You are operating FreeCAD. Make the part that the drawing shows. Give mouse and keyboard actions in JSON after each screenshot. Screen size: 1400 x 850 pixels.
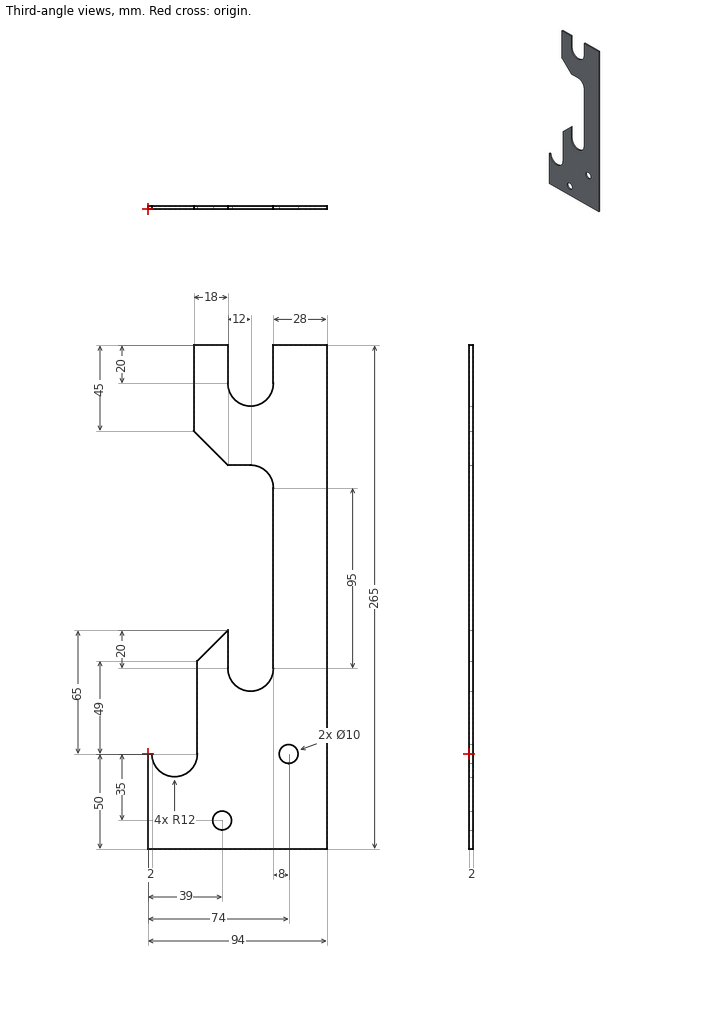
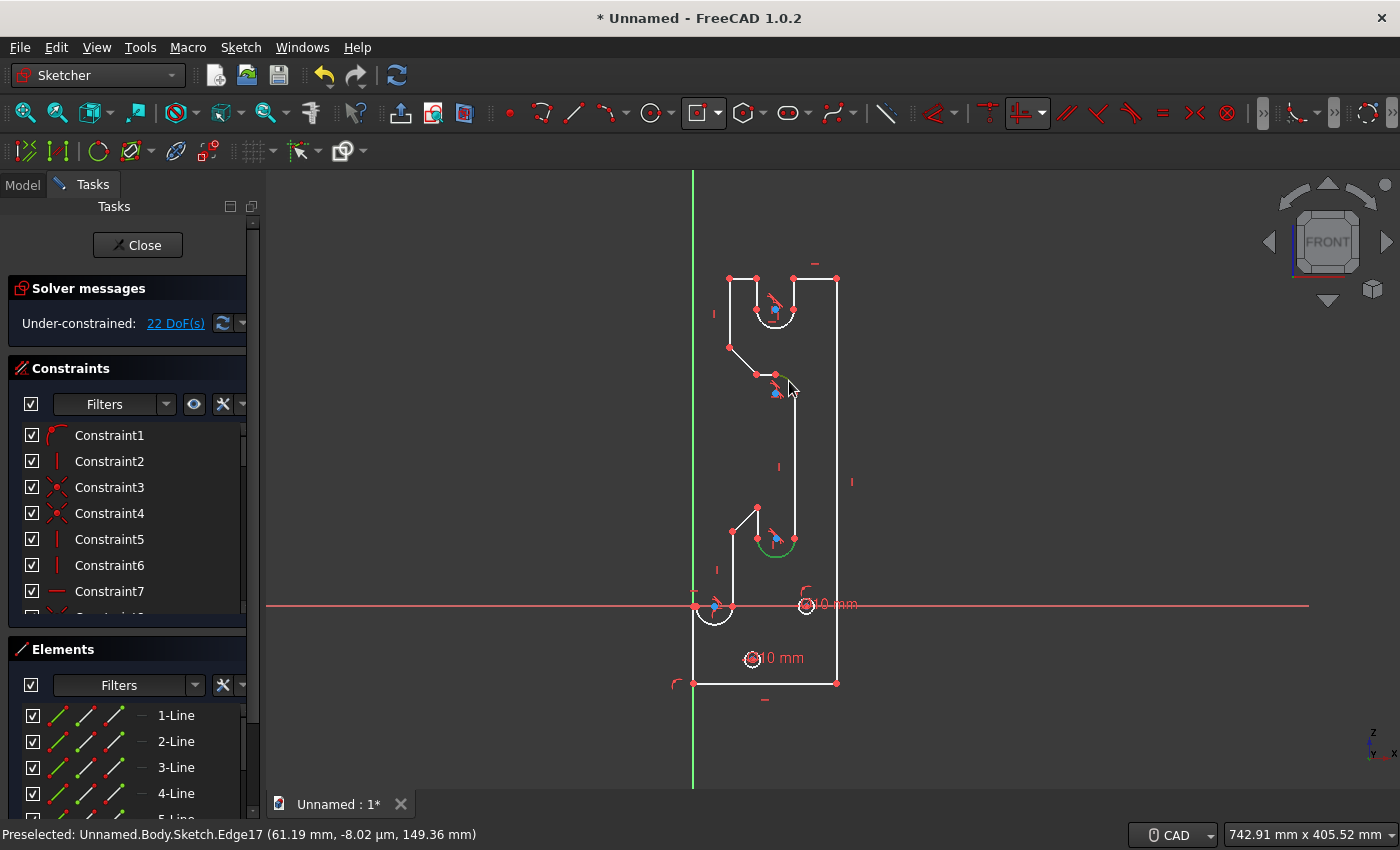
{"action": "left_click", "coordinate": [765, 325]}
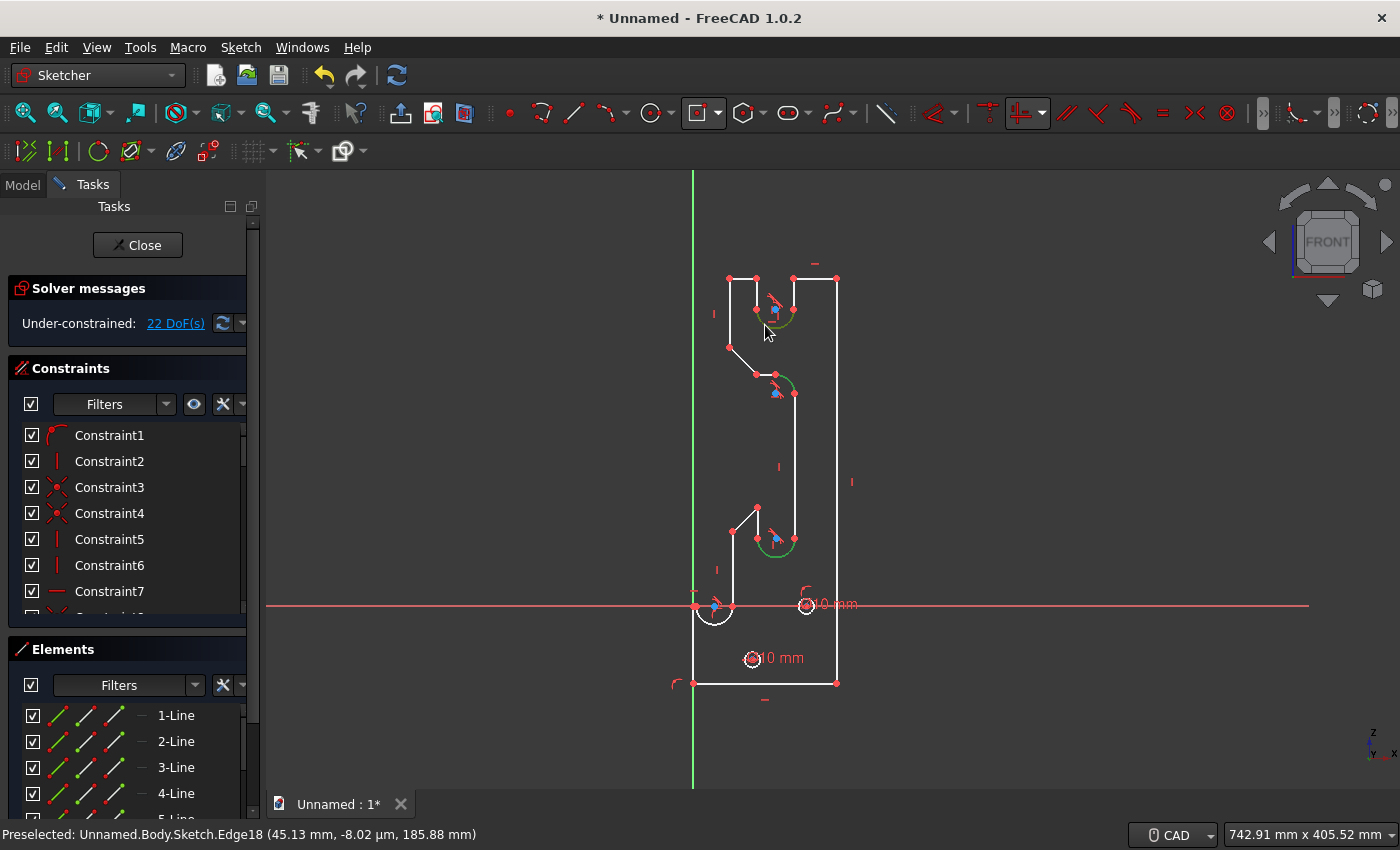
{"action": "scroll", "coordinate": [704, 621], "scroll_direction": "up", "scroll_amount": 2}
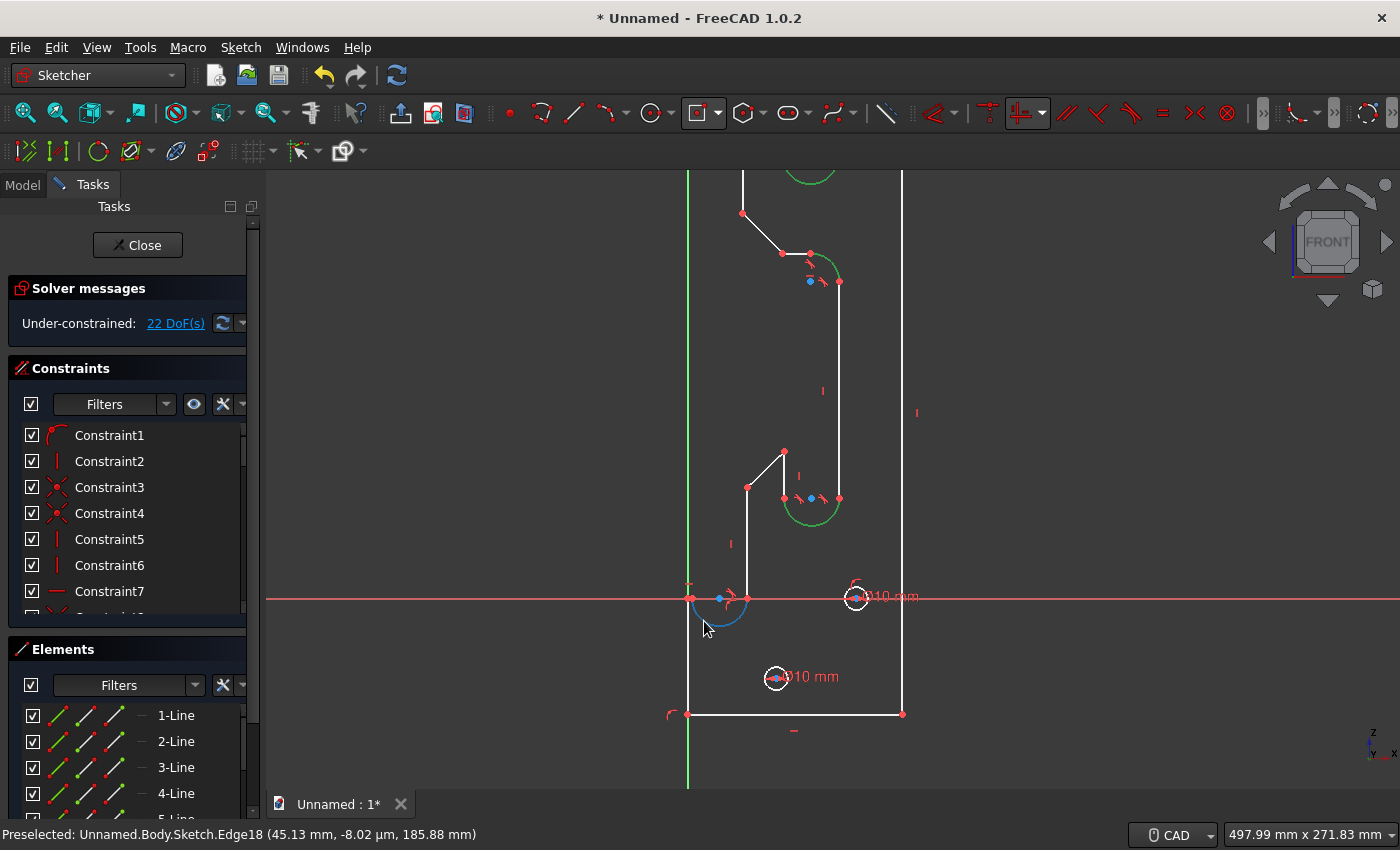
{"action": "left_click", "coordinate": [703, 621]}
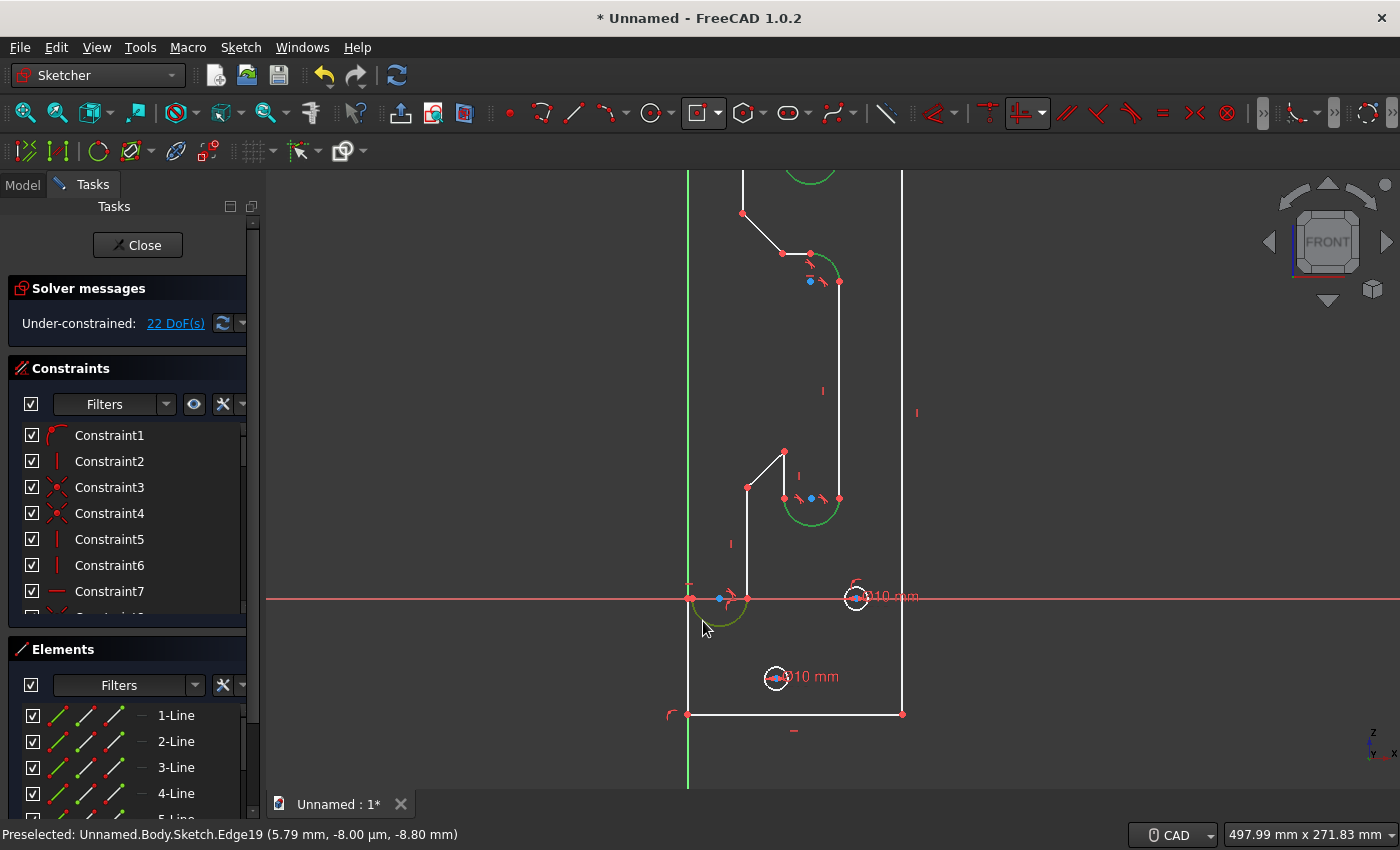
{"action": "key", "text": "e"}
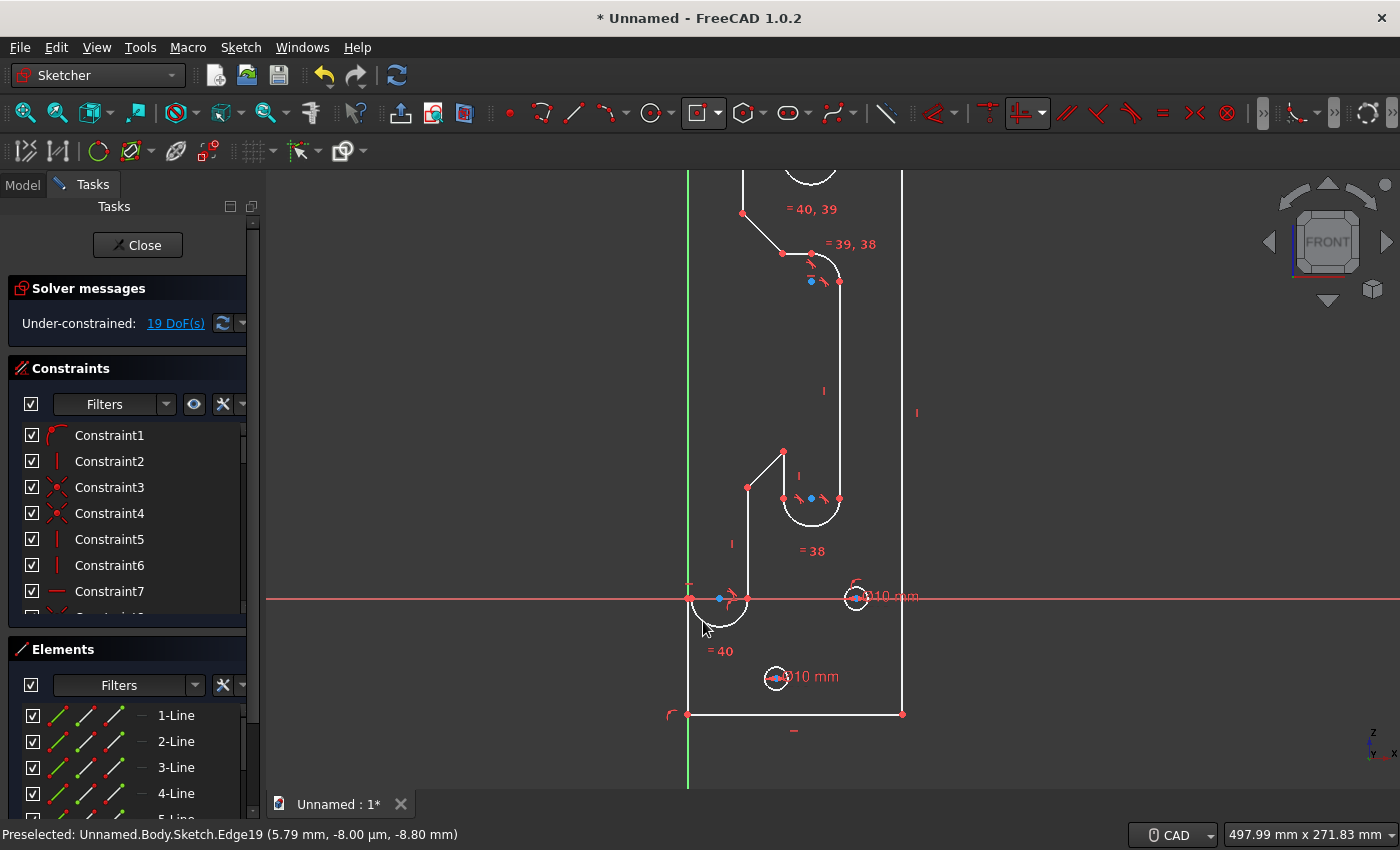
{"action": "key", "text": "d"}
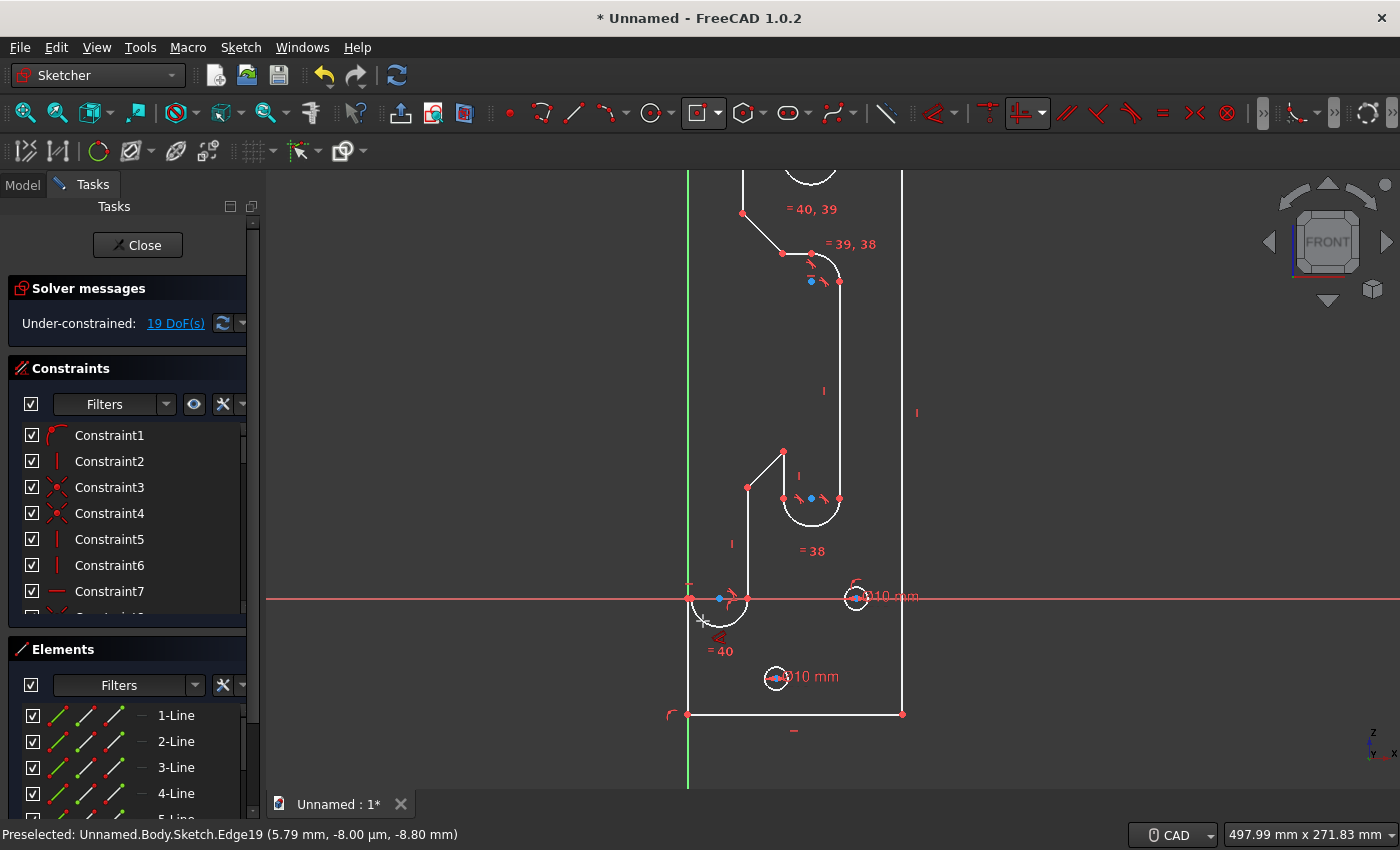
{"action": "scroll", "coordinate": [795, 521], "scroll_direction": "up", "scroll_amount": 2}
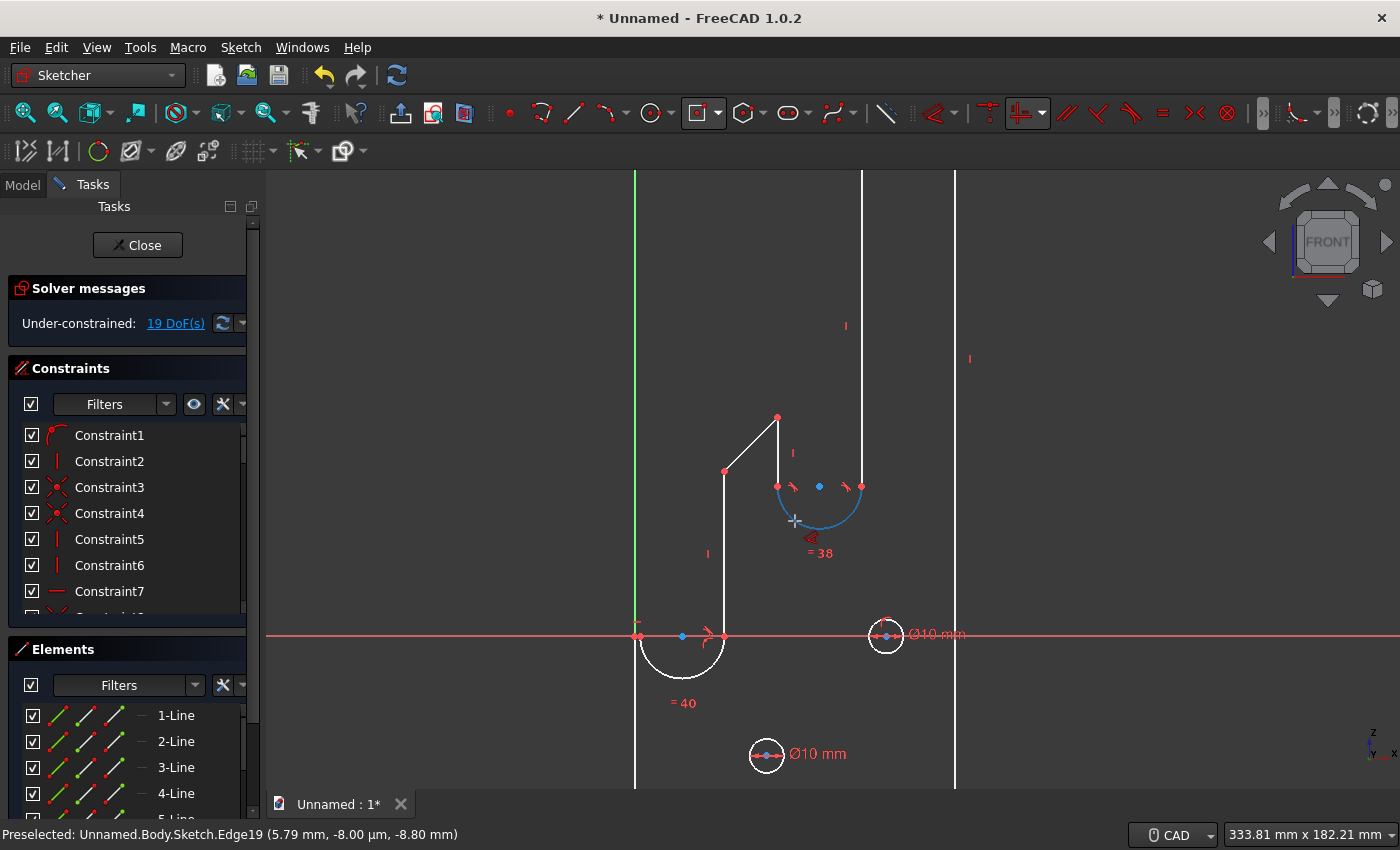
{"action": "left_click", "coordinate": [795, 521]}
{"action": "left_click", "coordinate": [776, 547]}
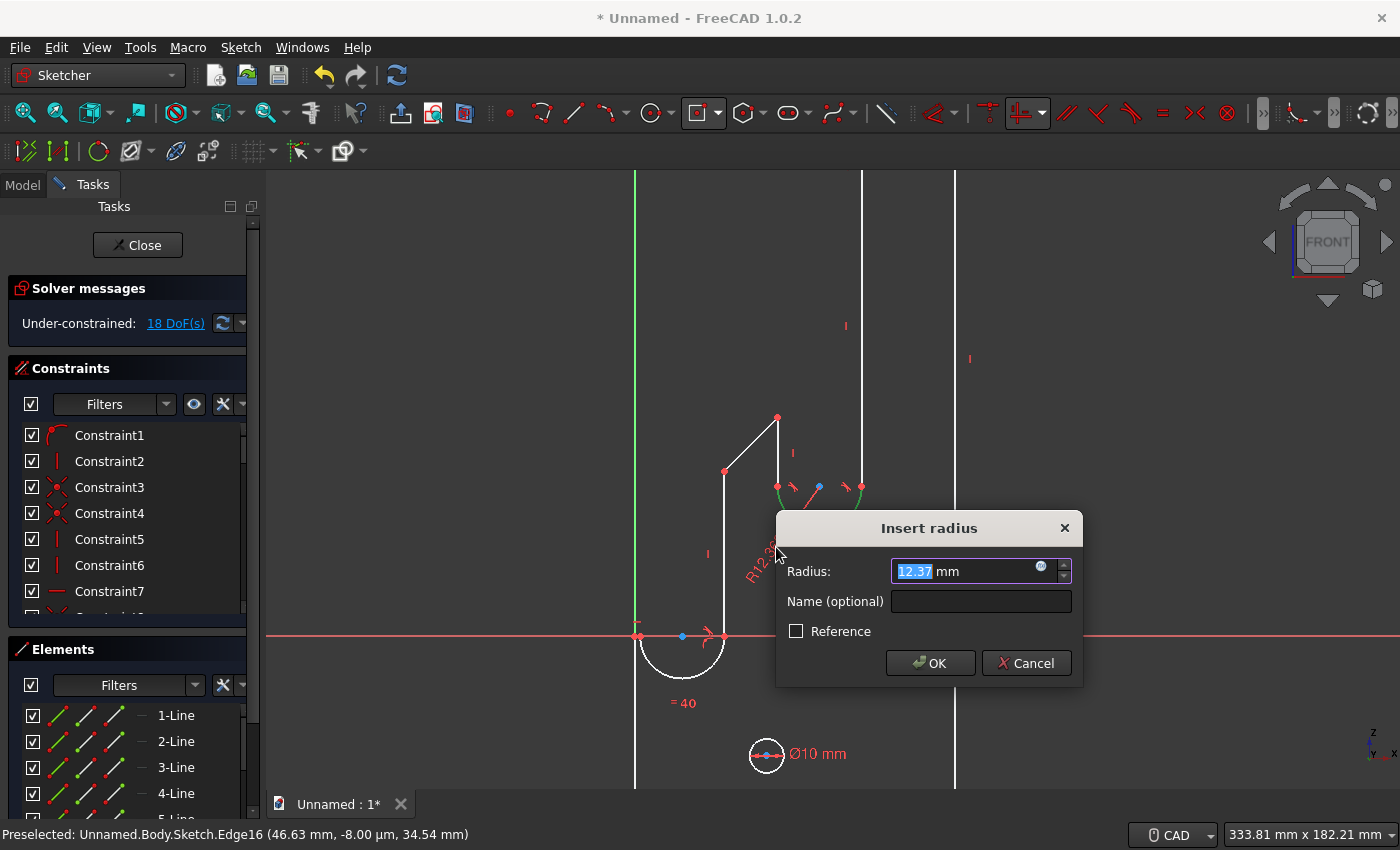
{"action": "type", "text": "12"}
{"action": "key", "text": "Return"}